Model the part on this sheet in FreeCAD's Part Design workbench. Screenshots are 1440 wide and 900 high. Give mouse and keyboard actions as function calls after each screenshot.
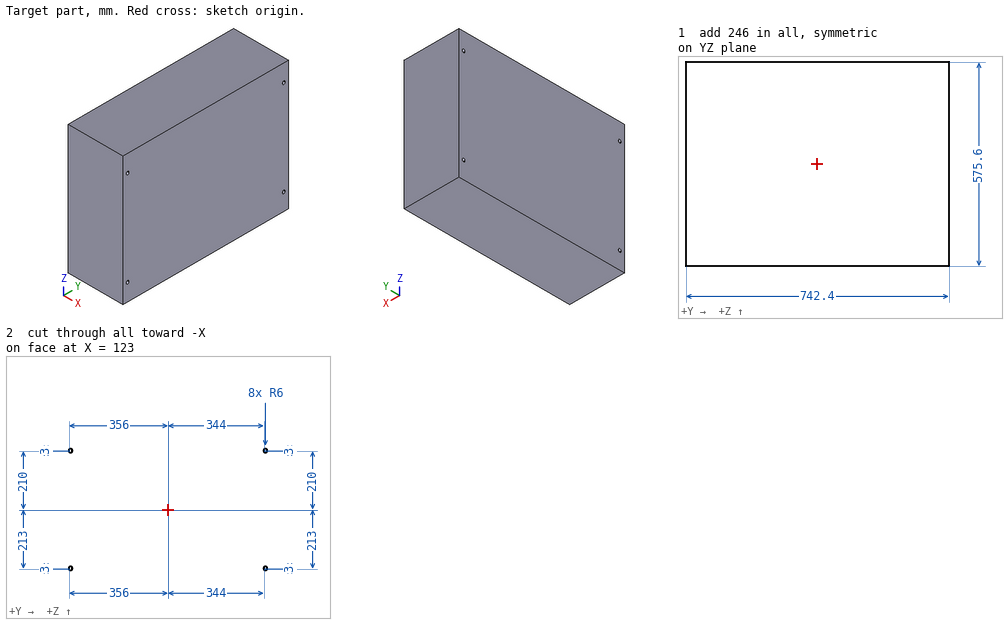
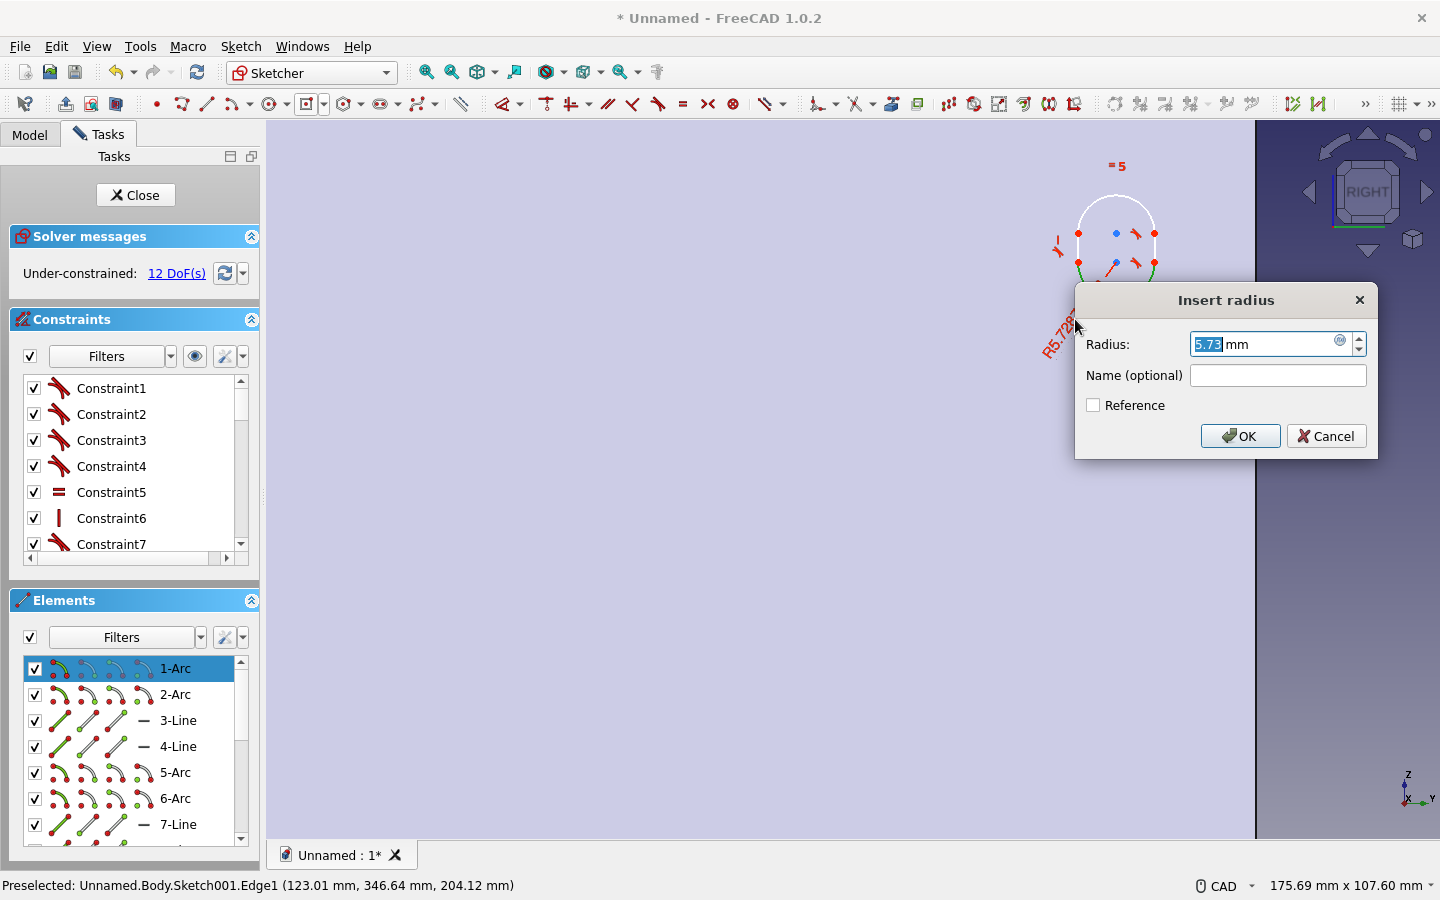
text(6)
key(Return)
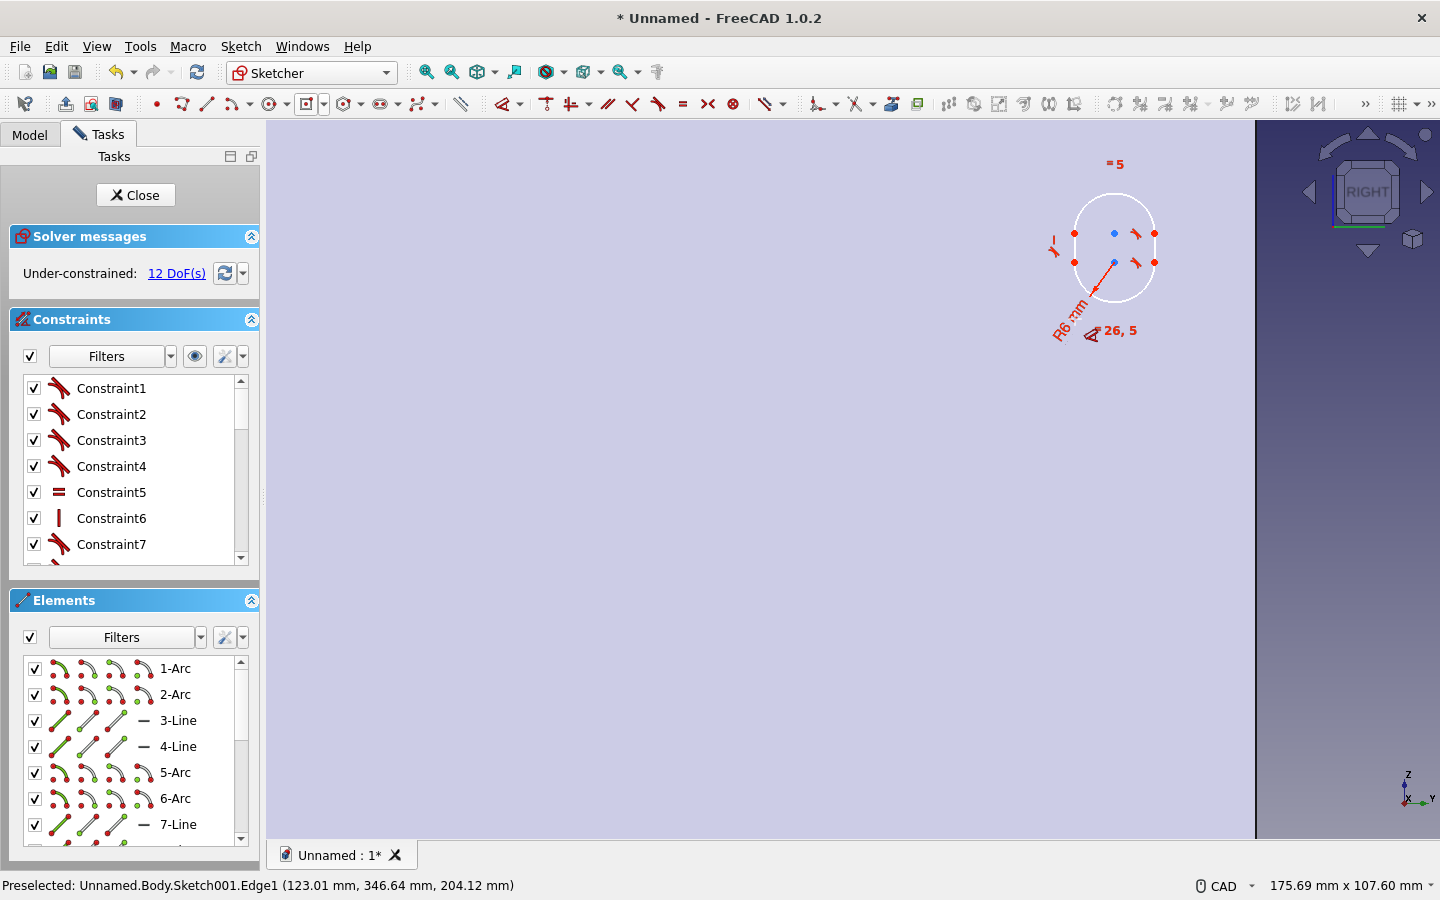
scroll(1075, 251, up, 4)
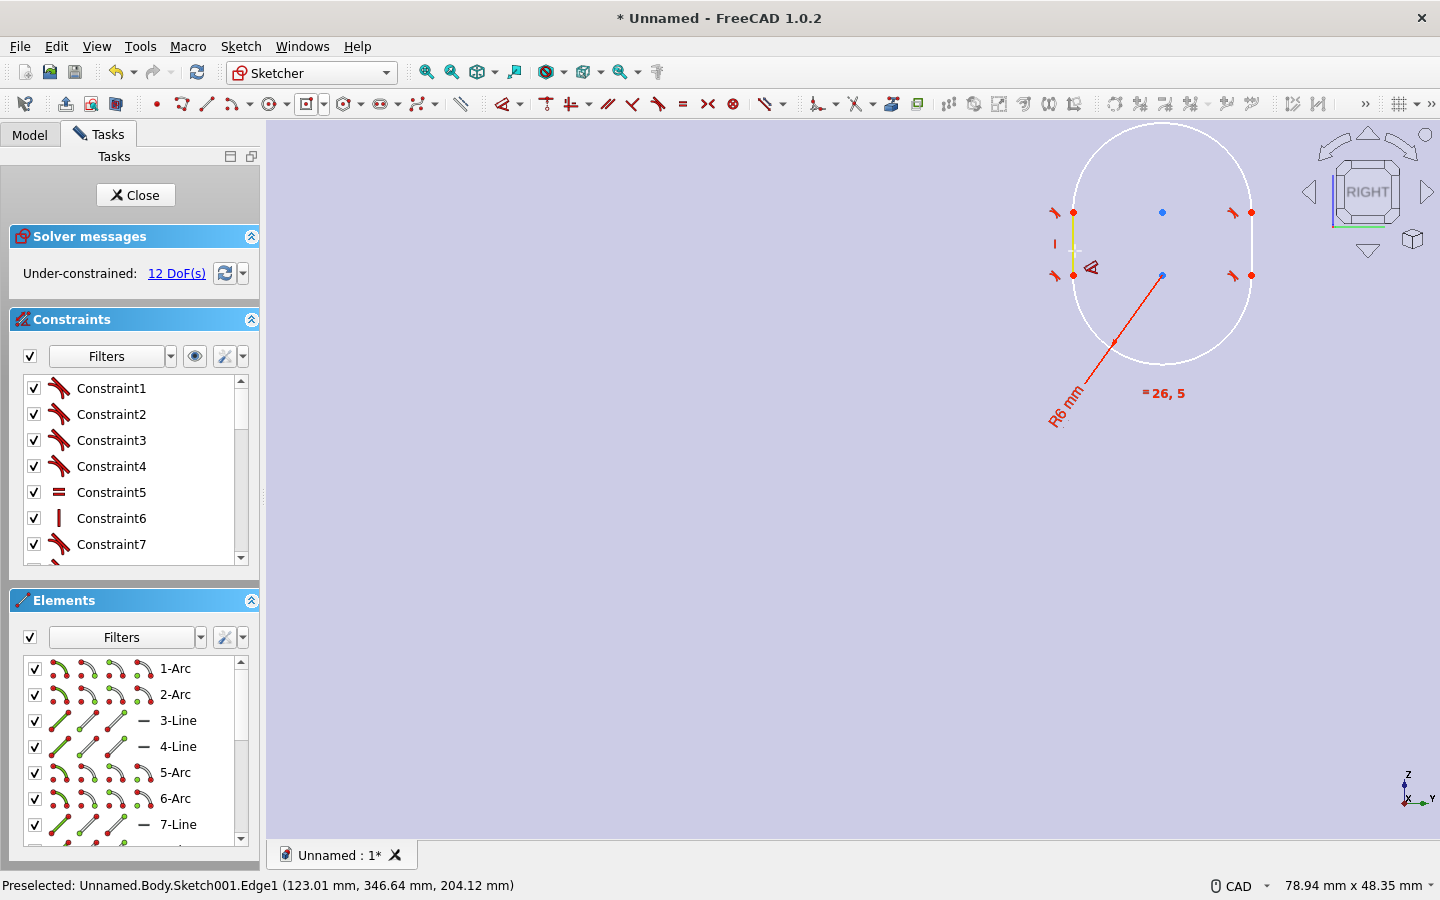
click(1073, 250)
click(1107, 244)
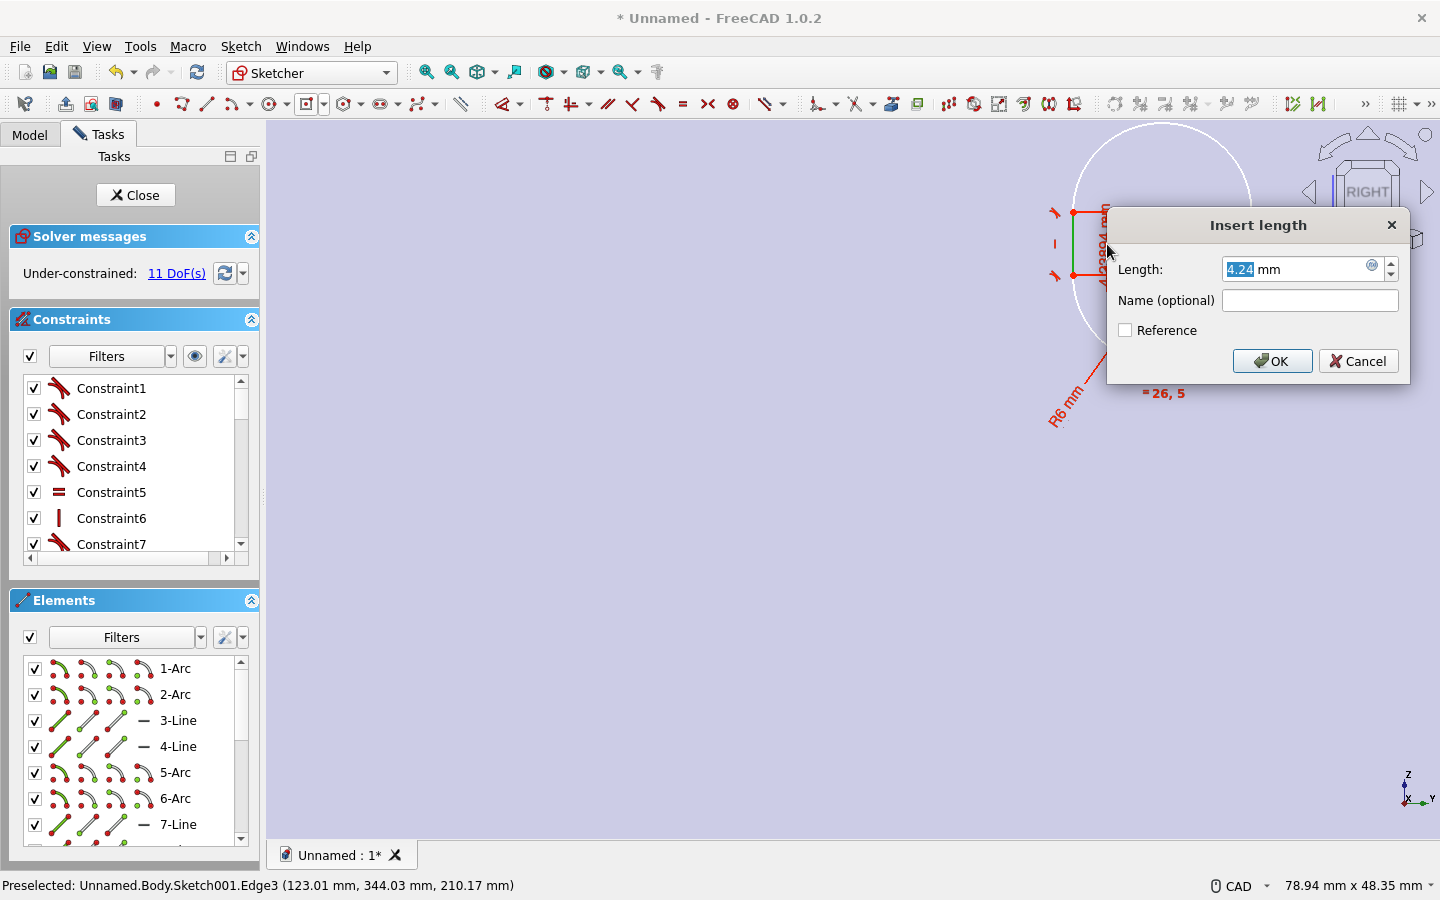
text(3)
key(Return)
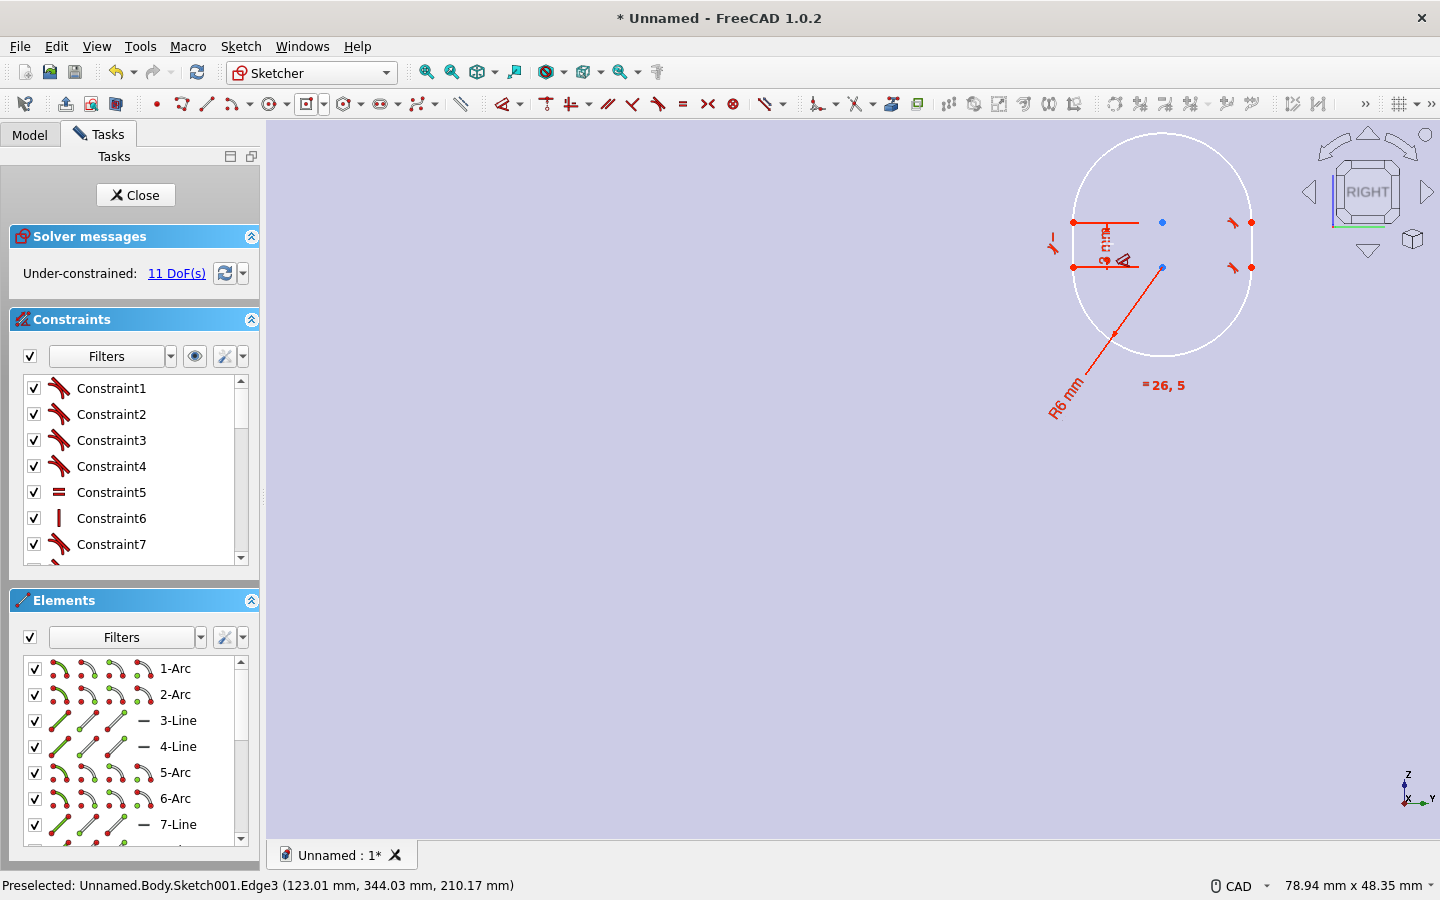
scroll(1097, 292, down, 14)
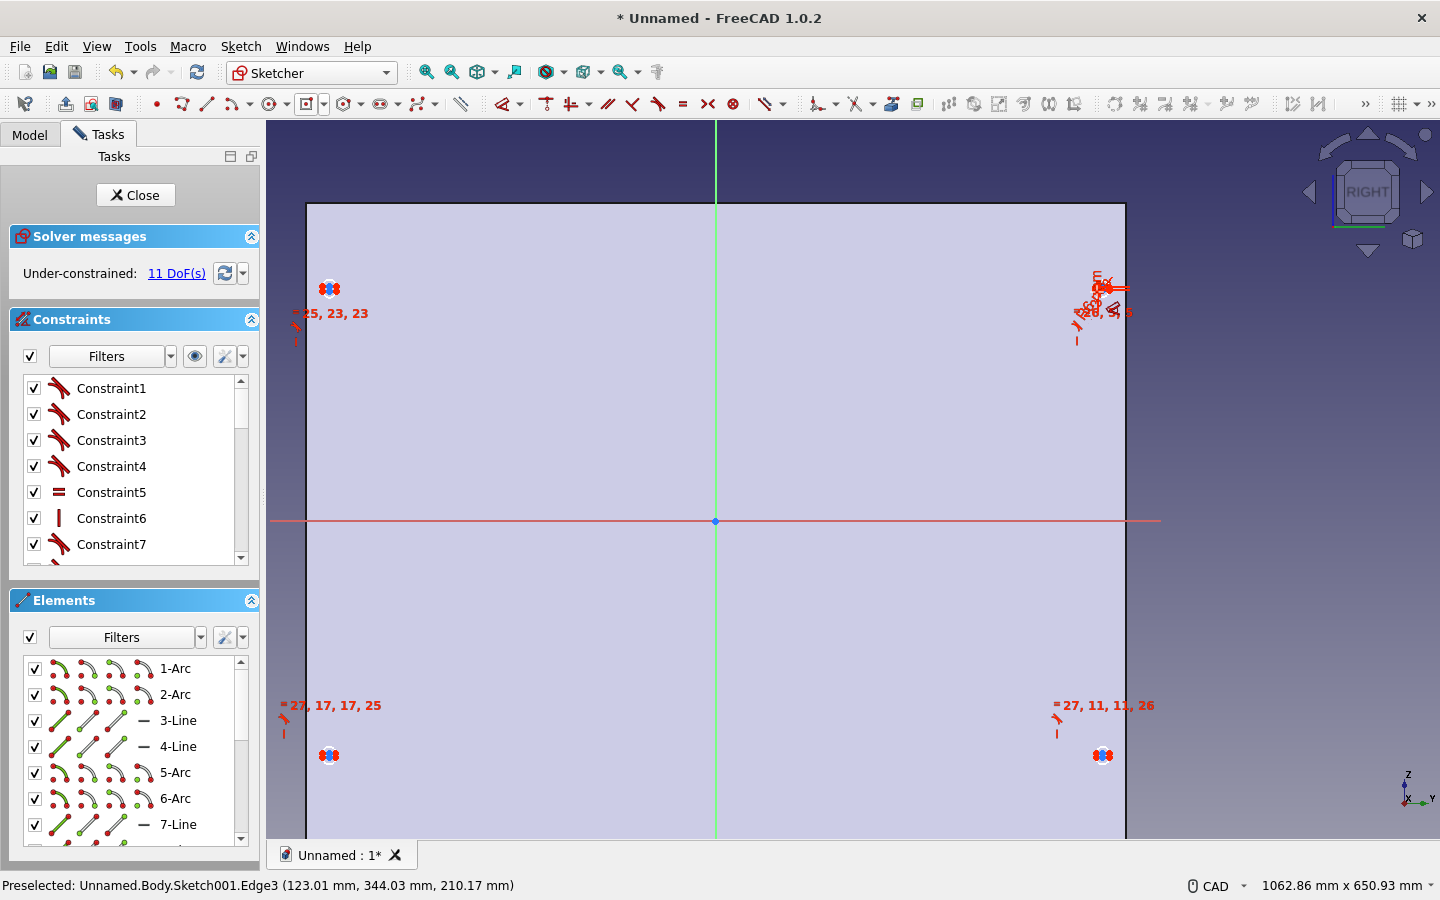
scroll(1096, 672, up, 14)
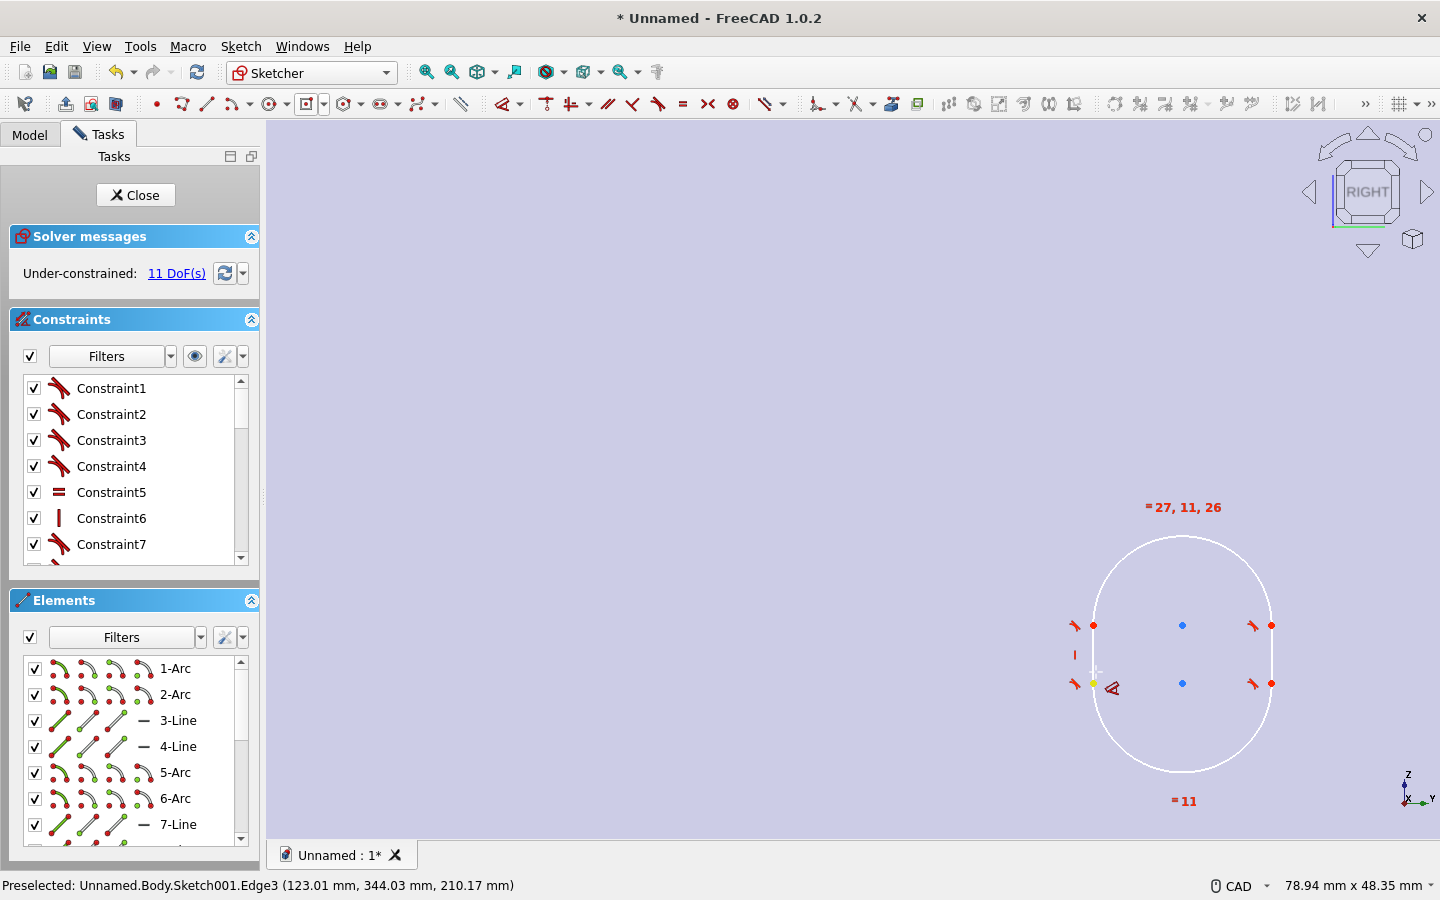
click(1093, 666)
click(1127, 654)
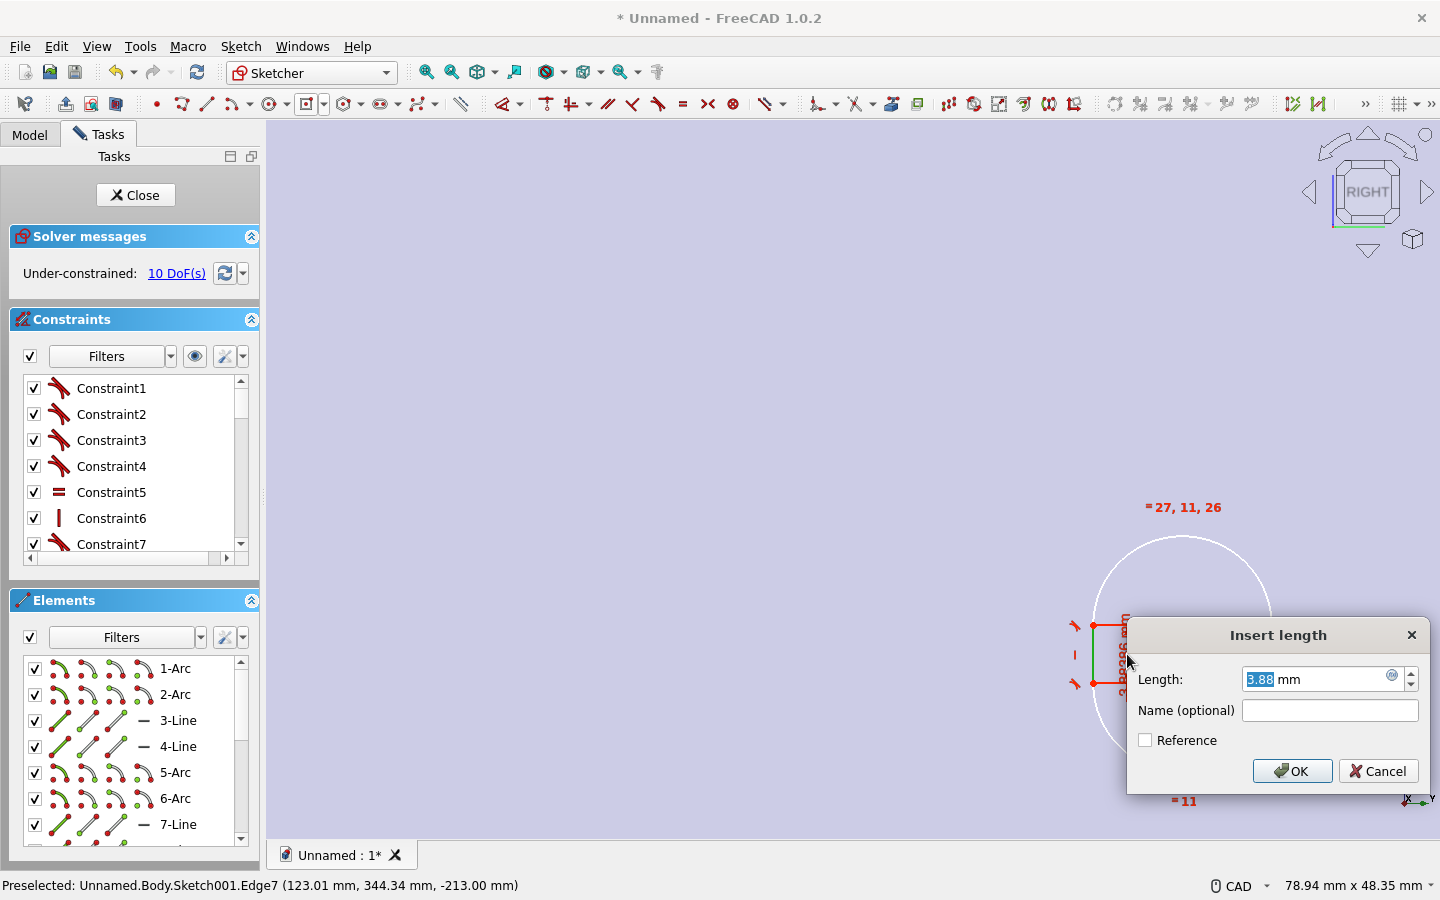
text(3)
key(Return)